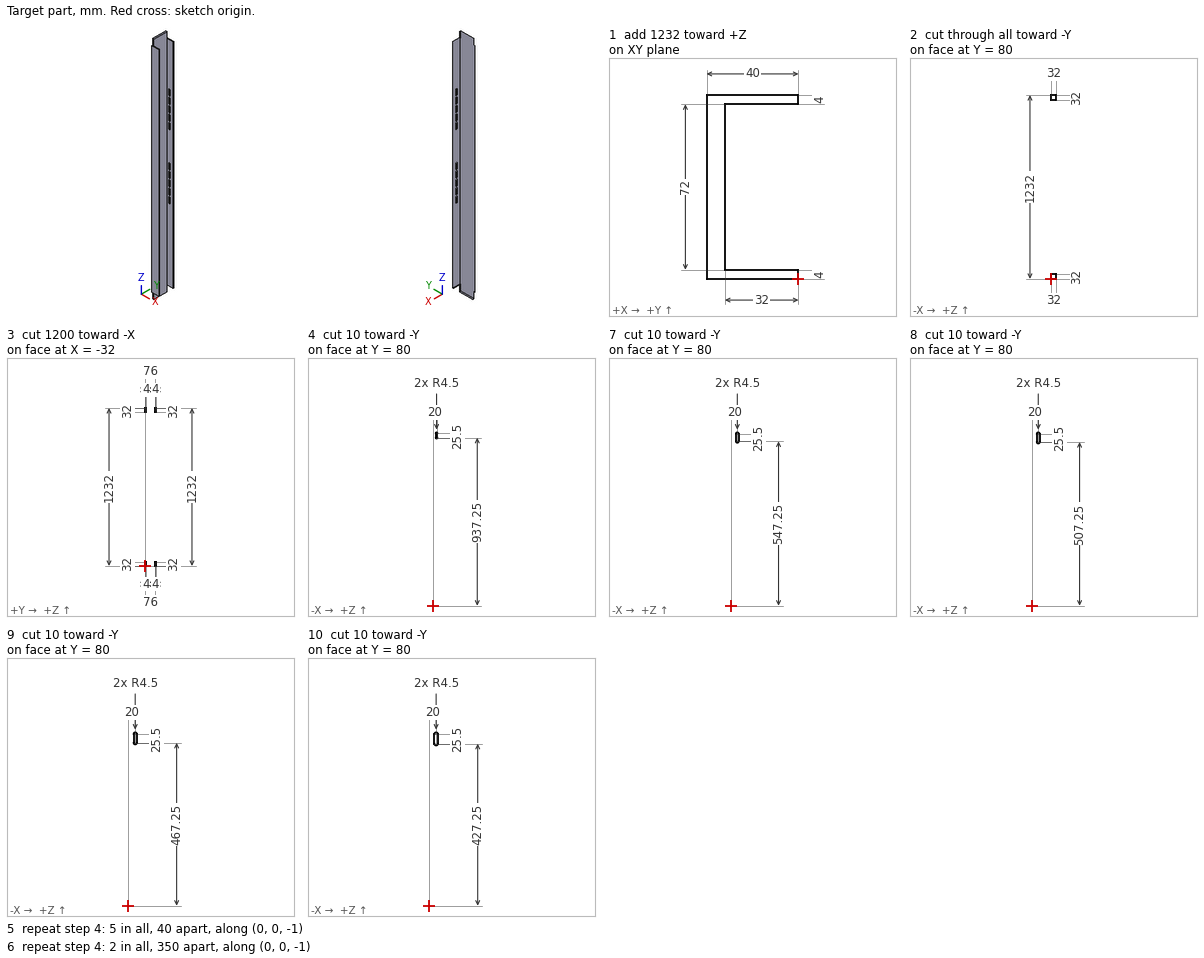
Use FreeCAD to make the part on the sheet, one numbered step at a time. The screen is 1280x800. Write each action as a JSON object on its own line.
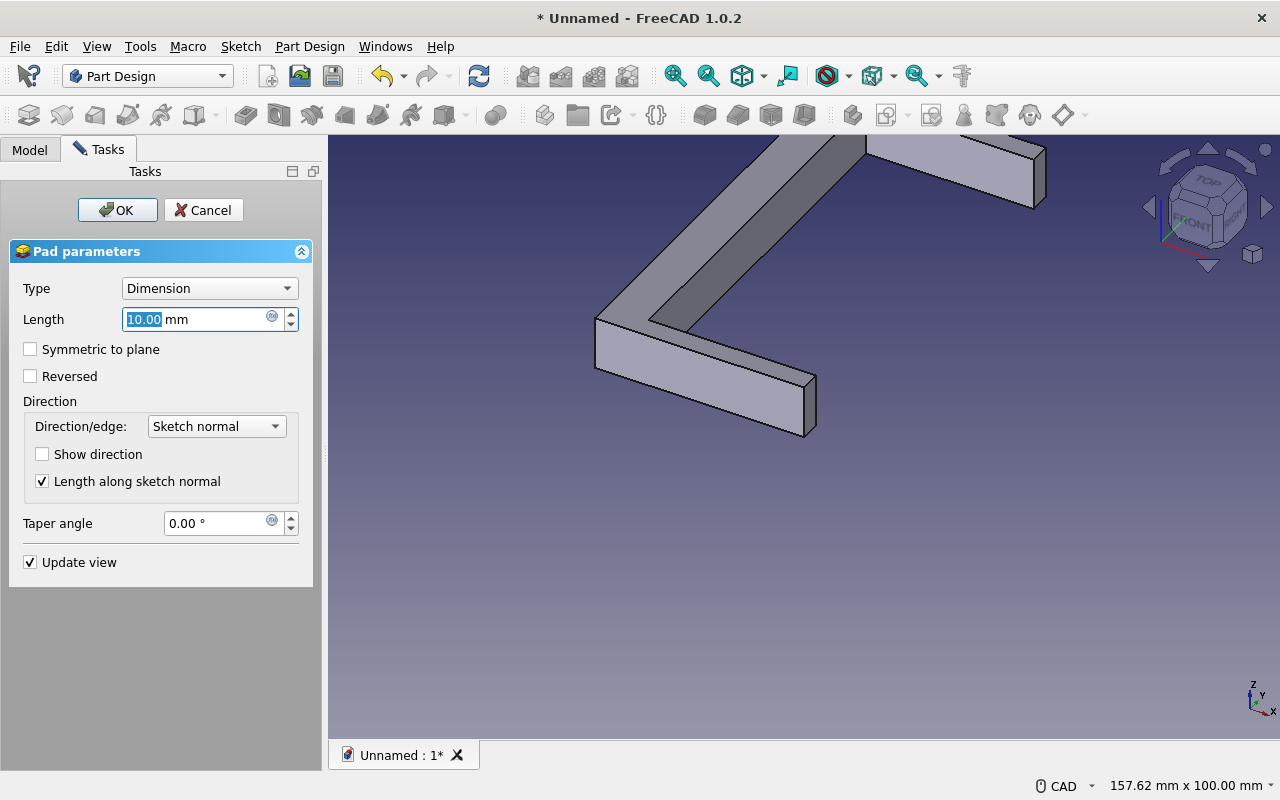
{"action": "type", "text": "1232"}
{"action": "key", "text": "Tab"}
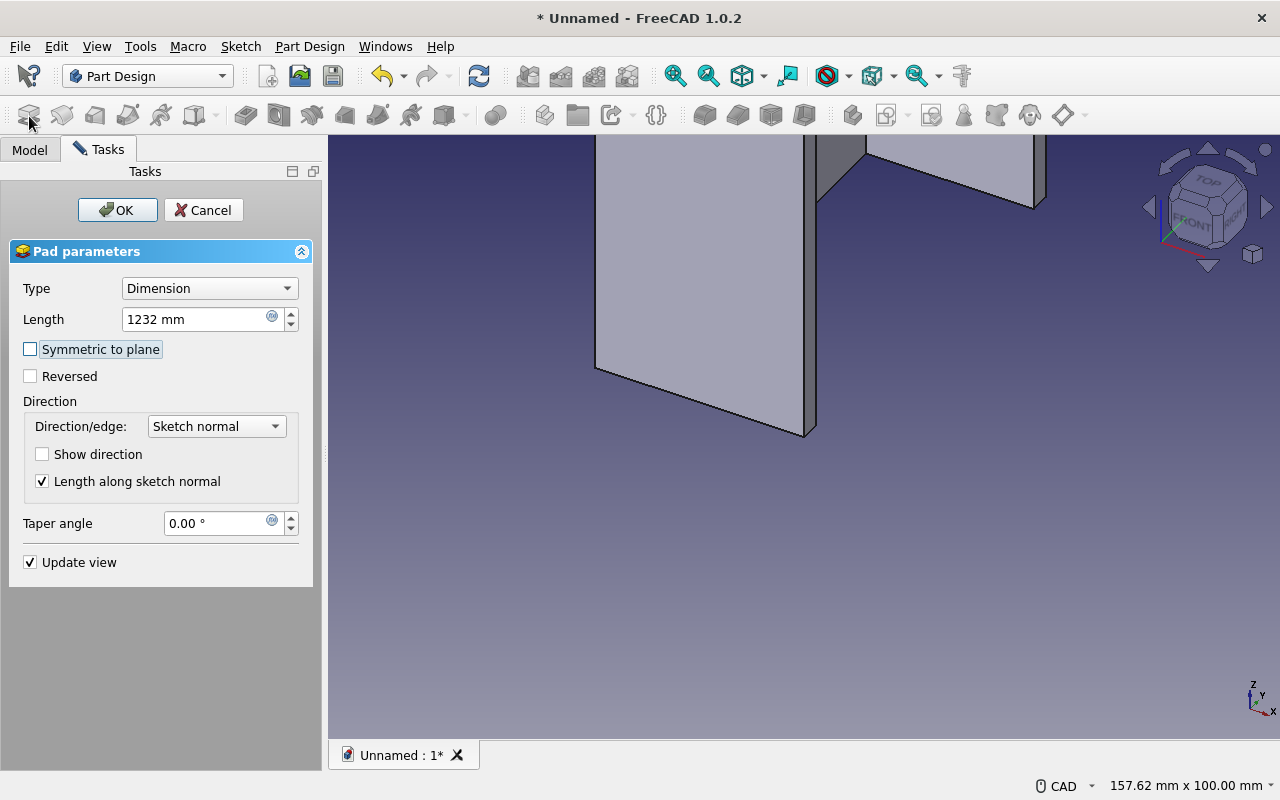
{"action": "left_click", "coordinate": [118, 210]}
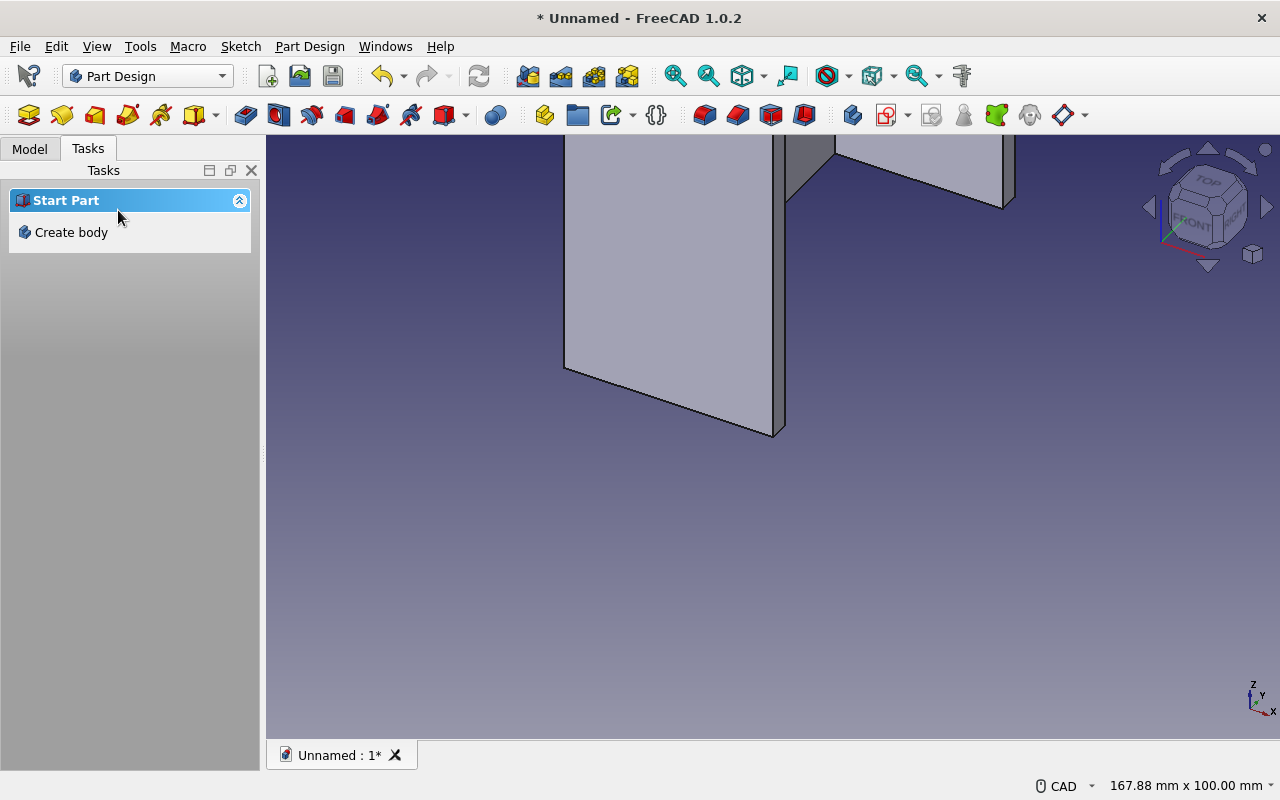
{"action": "key", "text": "v f"}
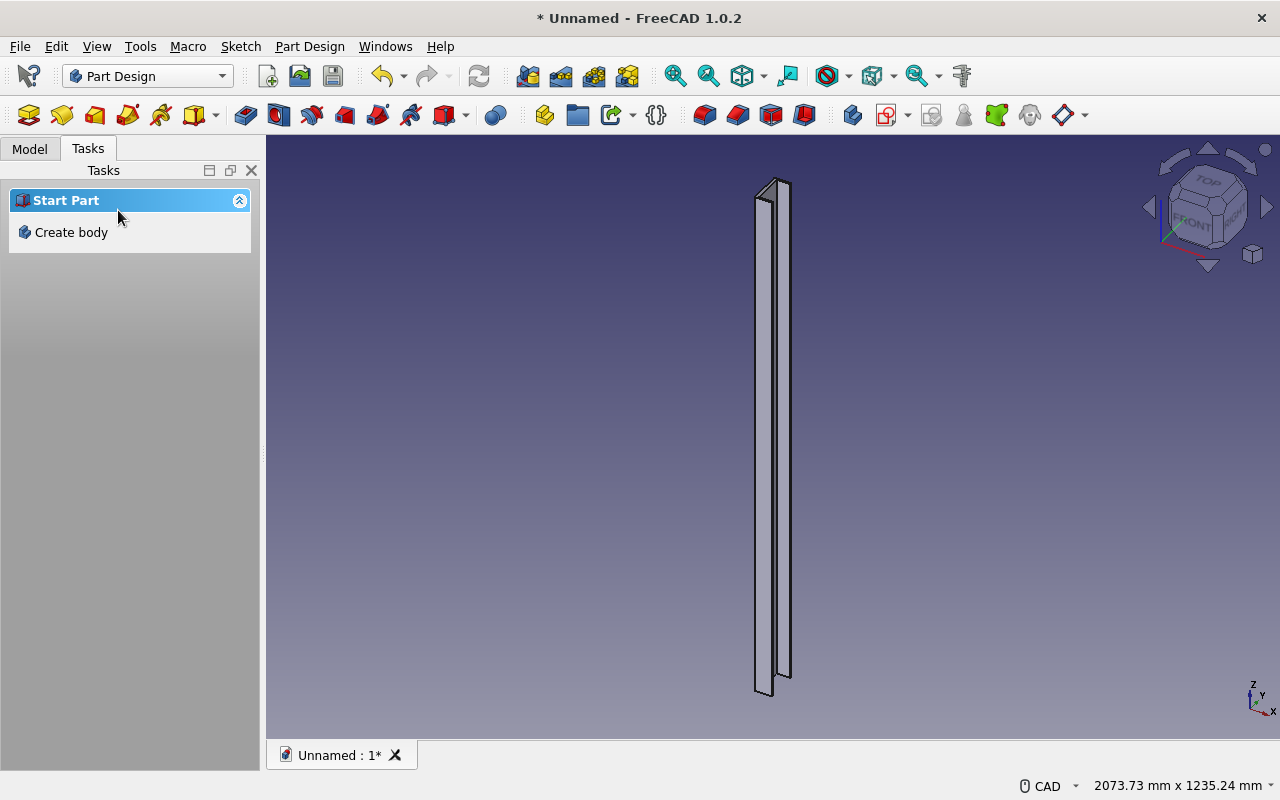
{"action": "key", "text": "4"}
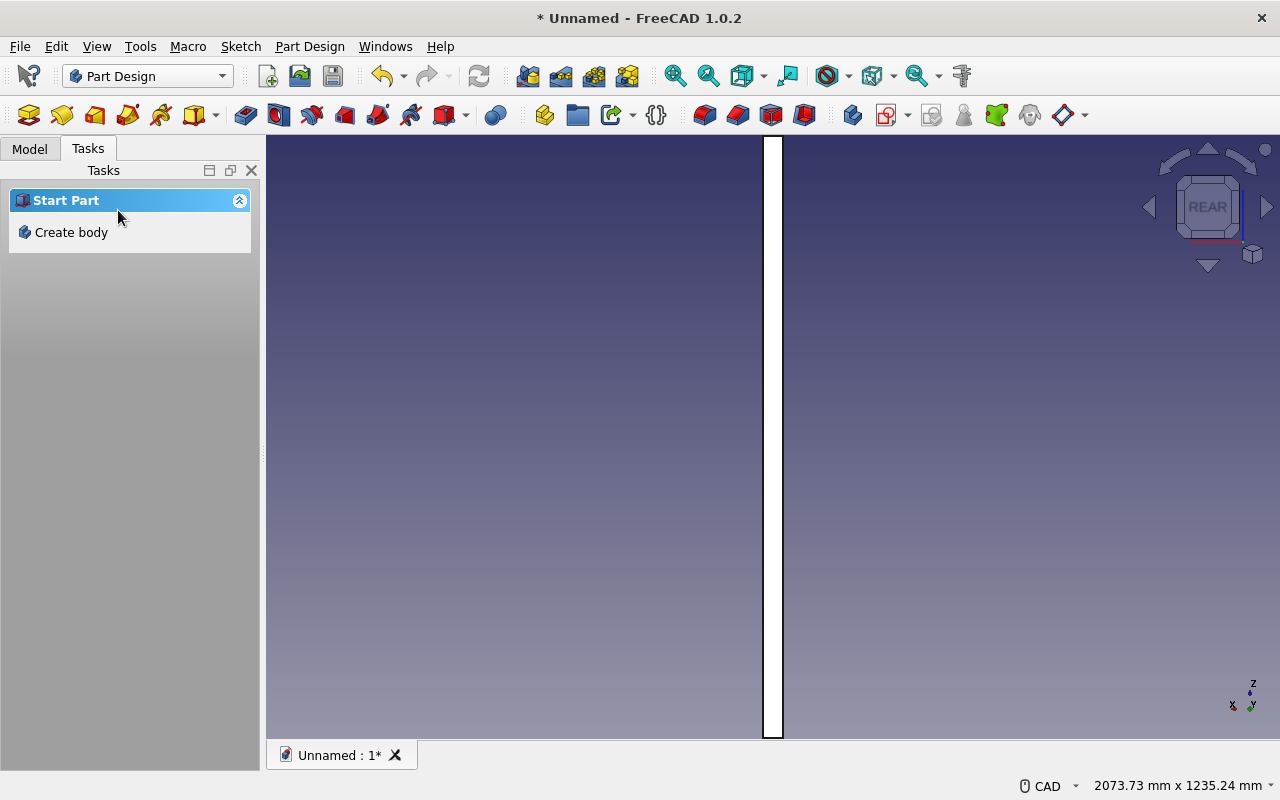
{"action": "left_click", "coordinate": [773, 178]}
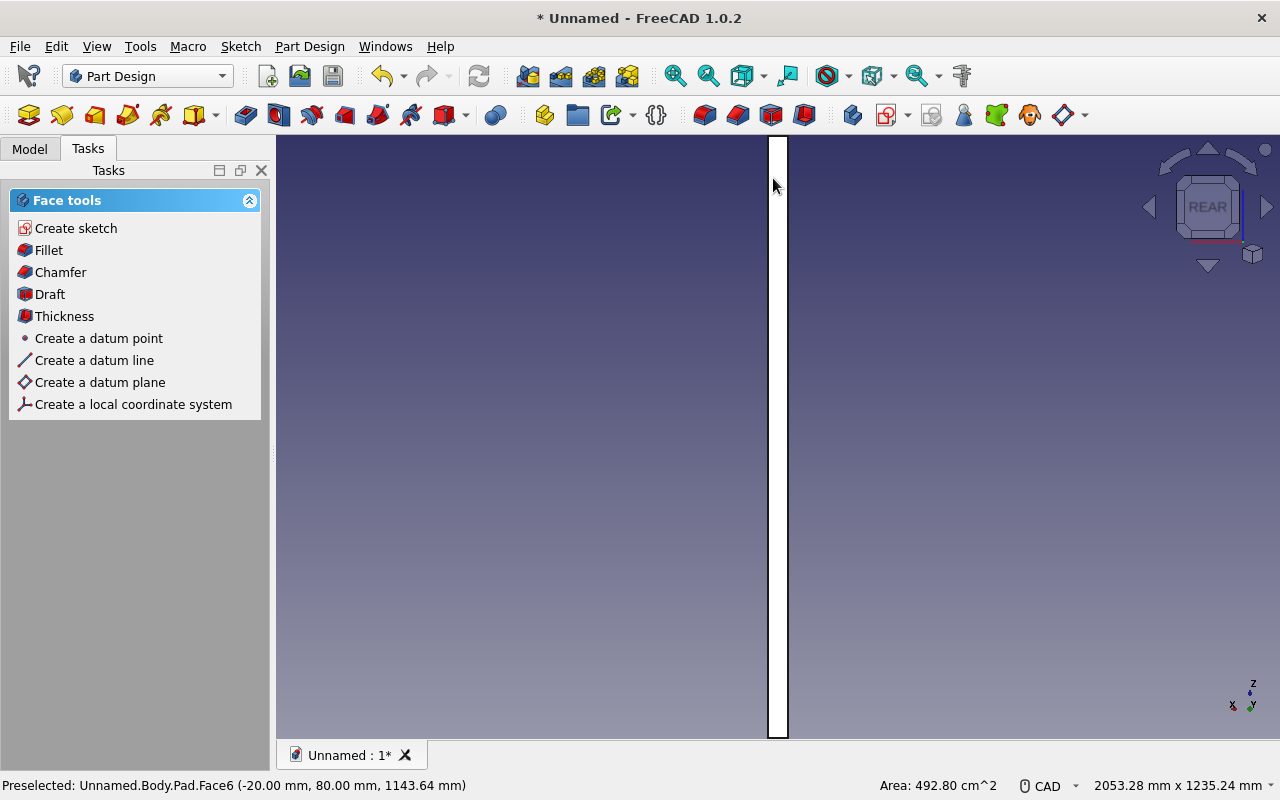
{"action": "left_click", "coordinate": [886, 116]}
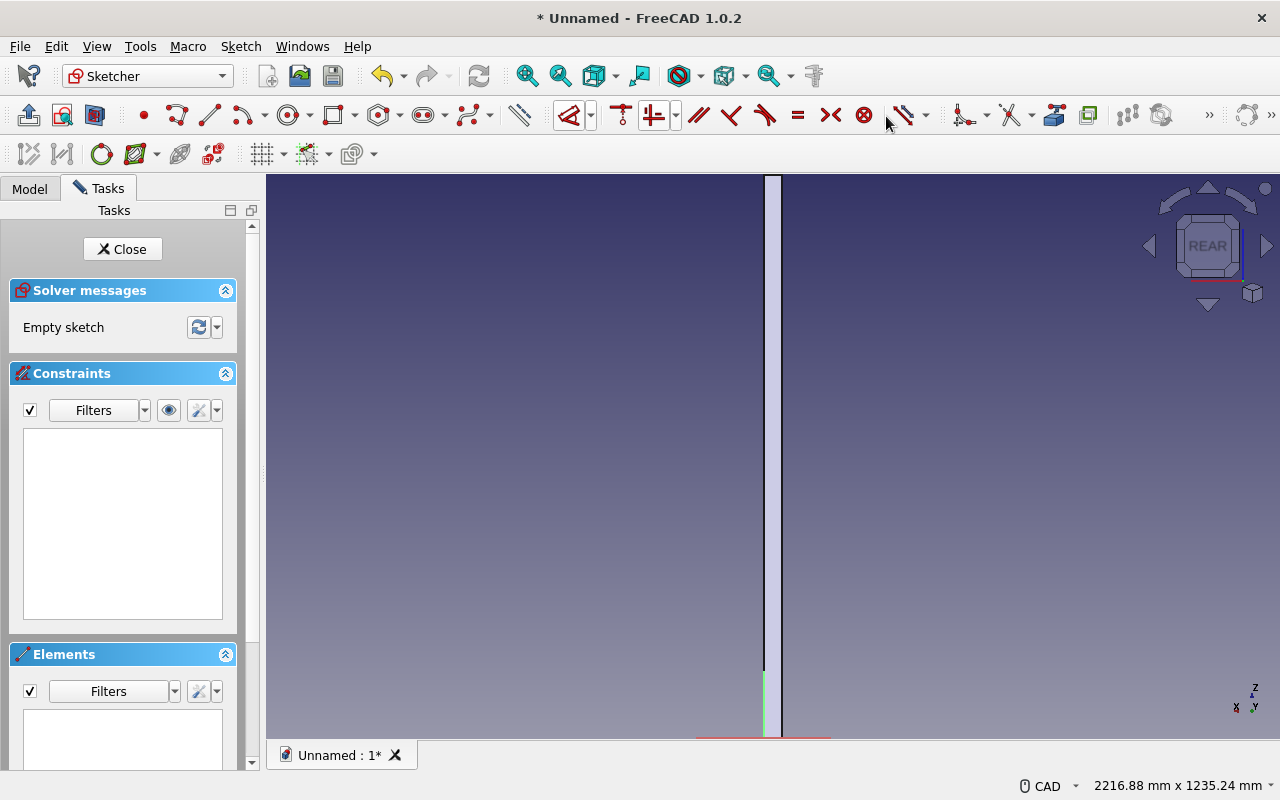
{"action": "scroll", "coordinate": [569, 457], "scroll_direction": "down", "scroll_amount": 2}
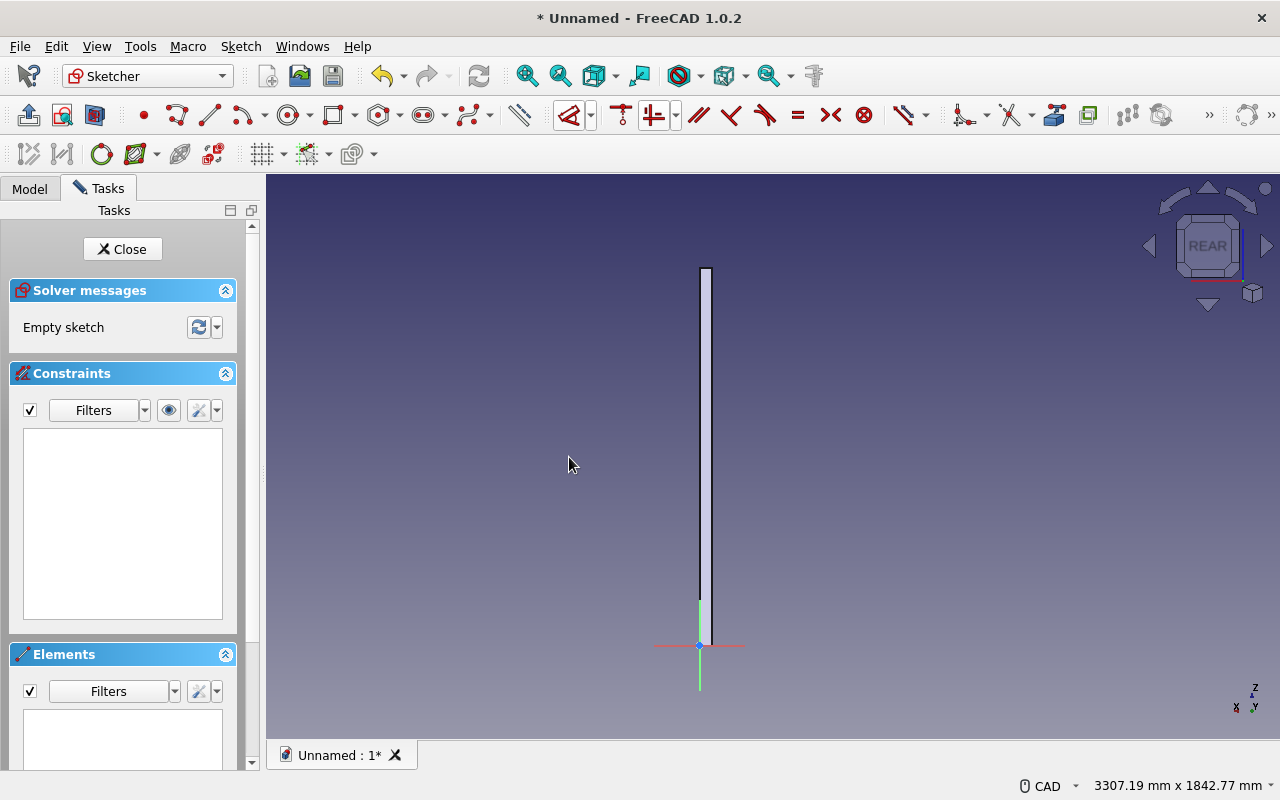
{"action": "left_click", "coordinate": [332, 116]}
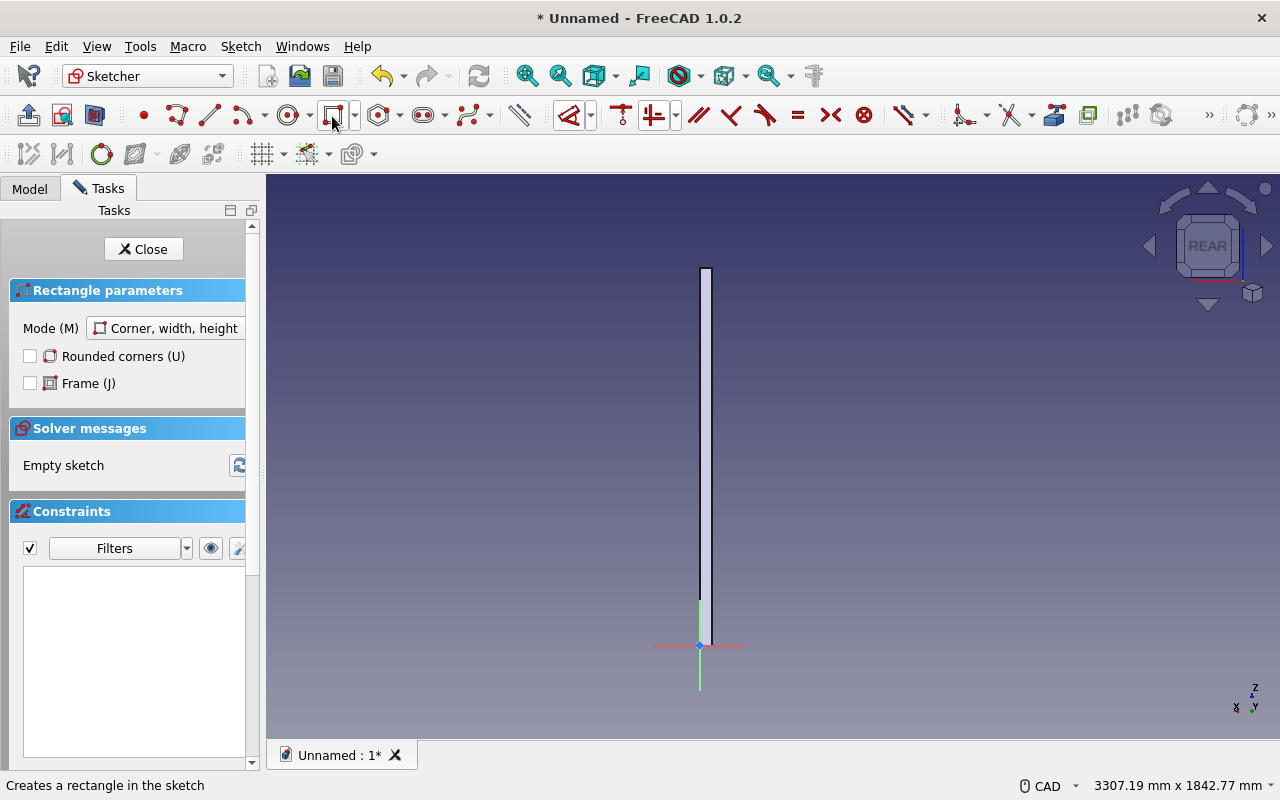
{"action": "scroll", "coordinate": [700, 646], "scroll_direction": "up", "scroll_amount": 3}